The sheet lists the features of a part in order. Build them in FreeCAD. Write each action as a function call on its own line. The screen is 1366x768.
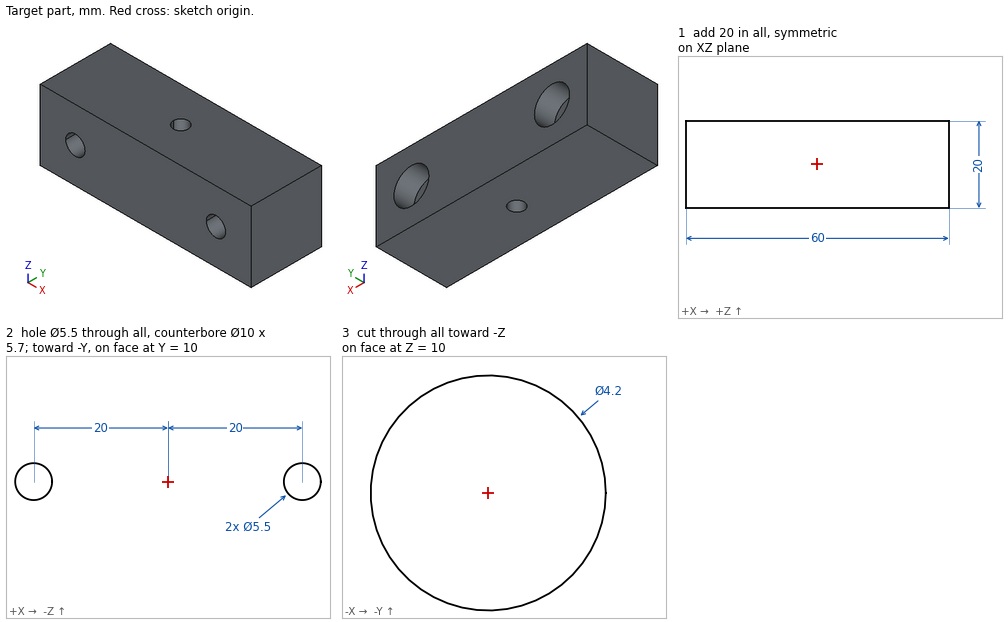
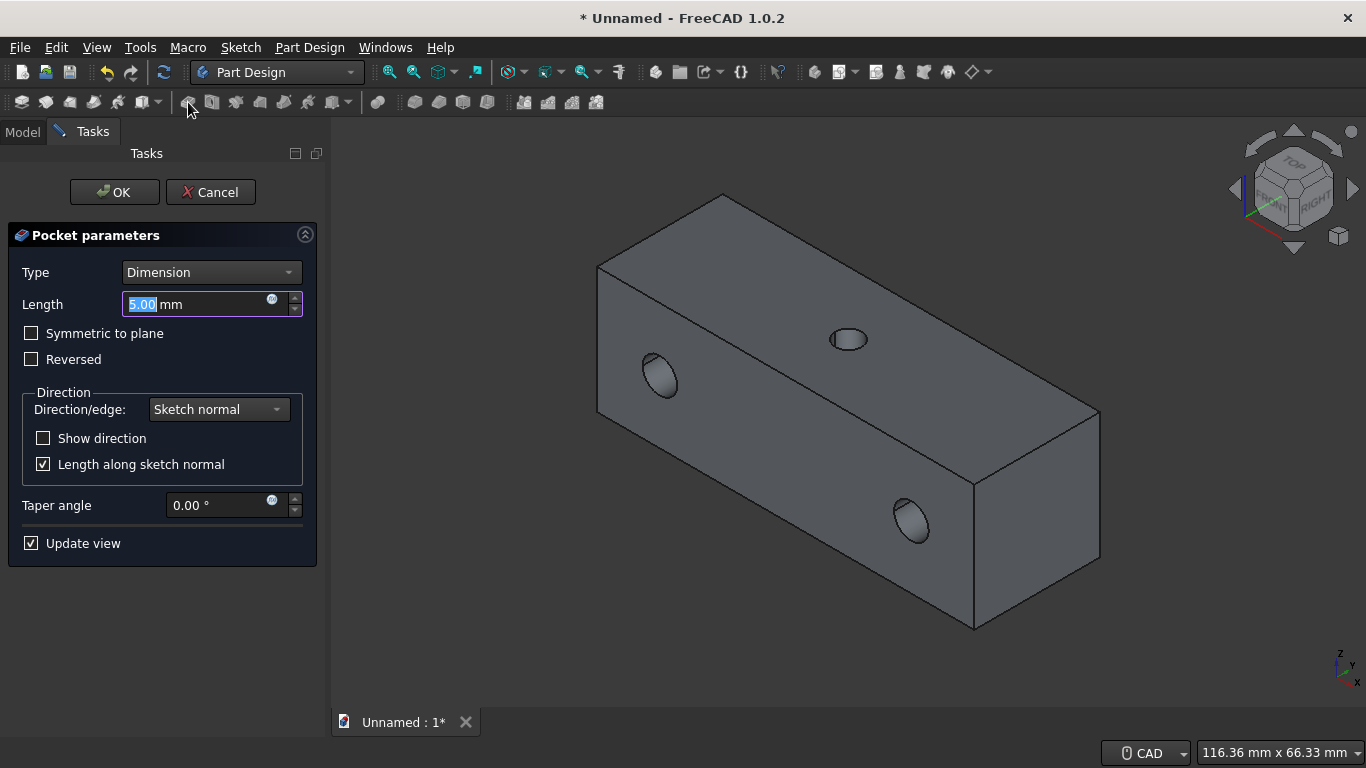
click(212, 272)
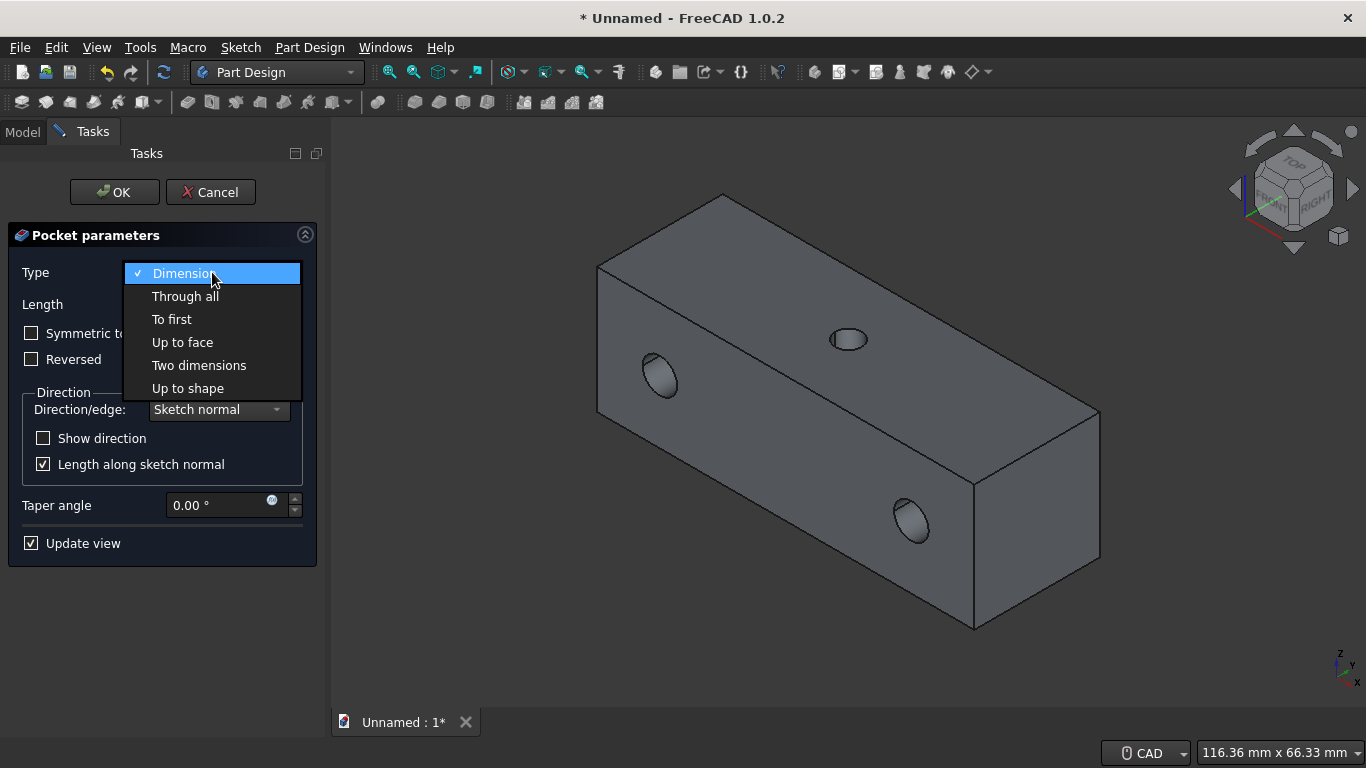
click(212, 296)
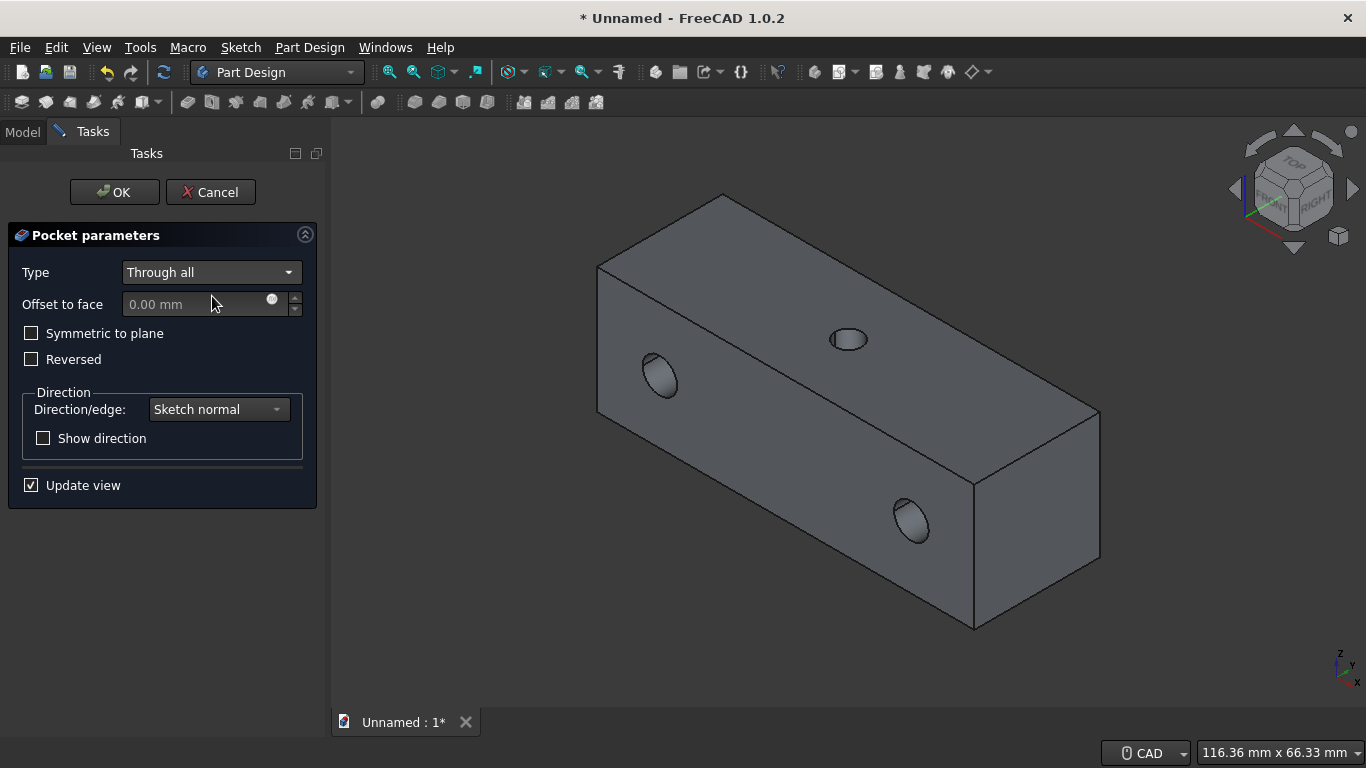
click(115, 192)